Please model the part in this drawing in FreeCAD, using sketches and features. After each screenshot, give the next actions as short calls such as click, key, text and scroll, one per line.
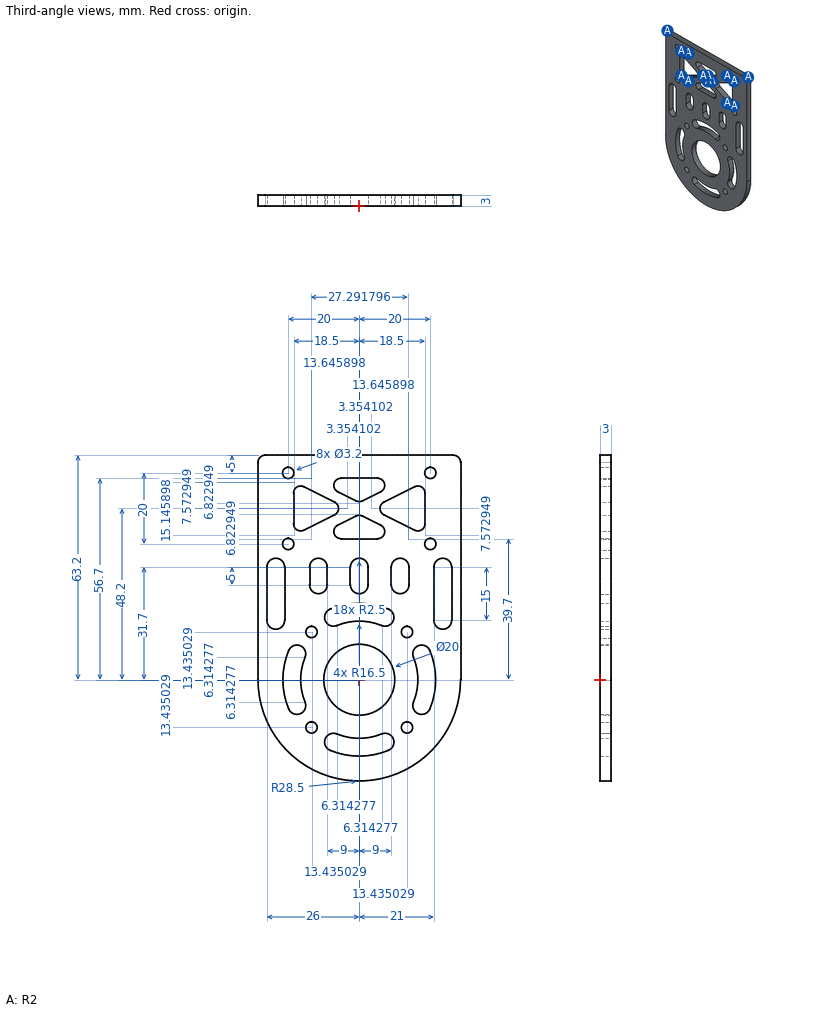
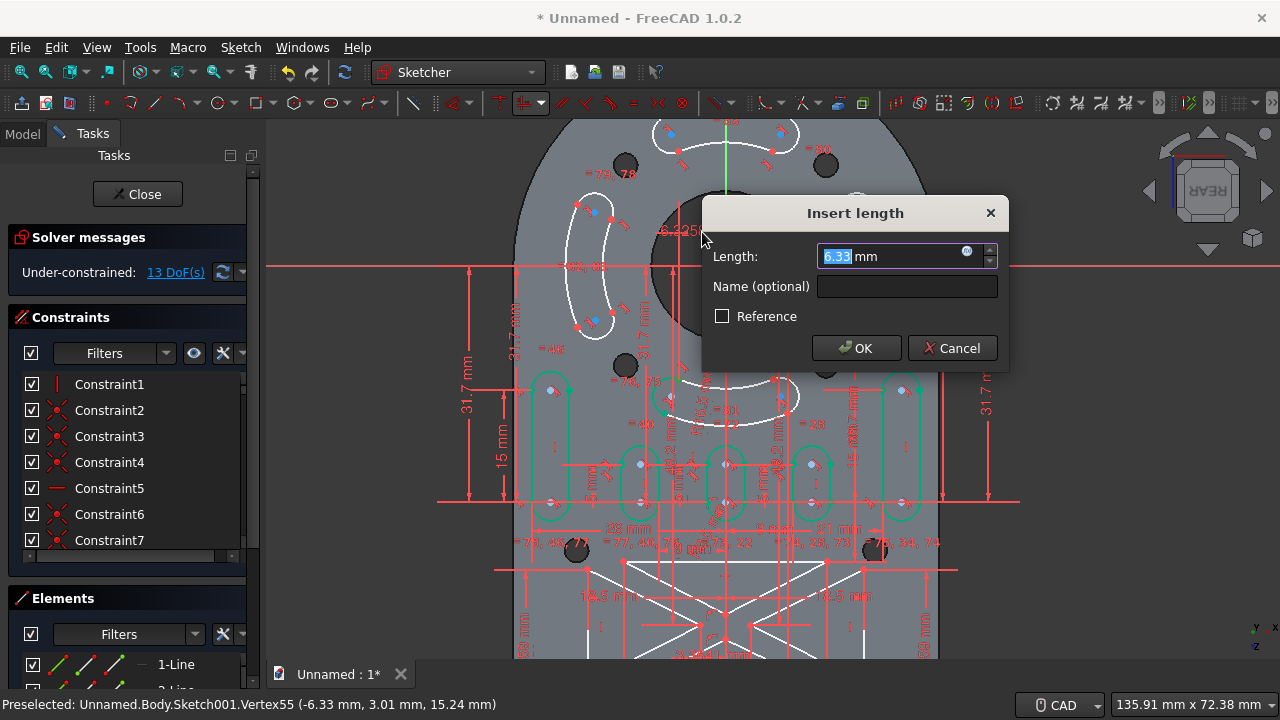
text(6.314277)
key(Return)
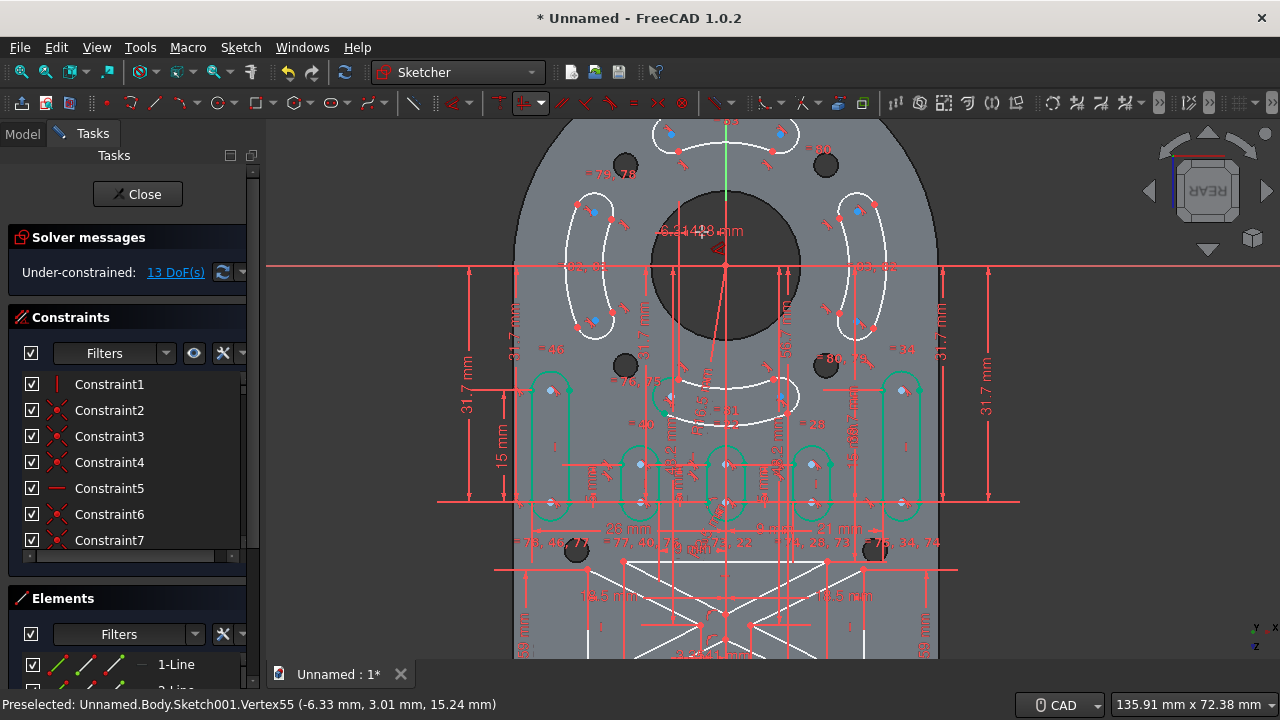
click(773, 379)
click(749, 208)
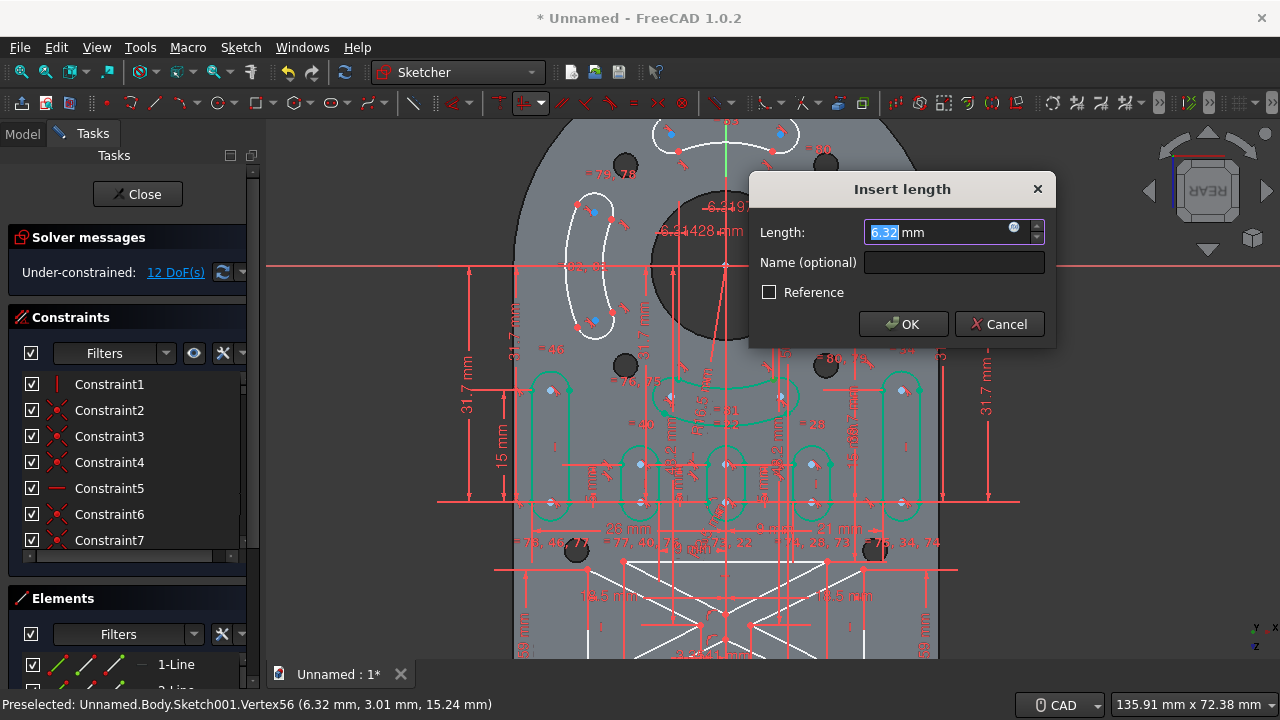
text(6.314277)
key(Return)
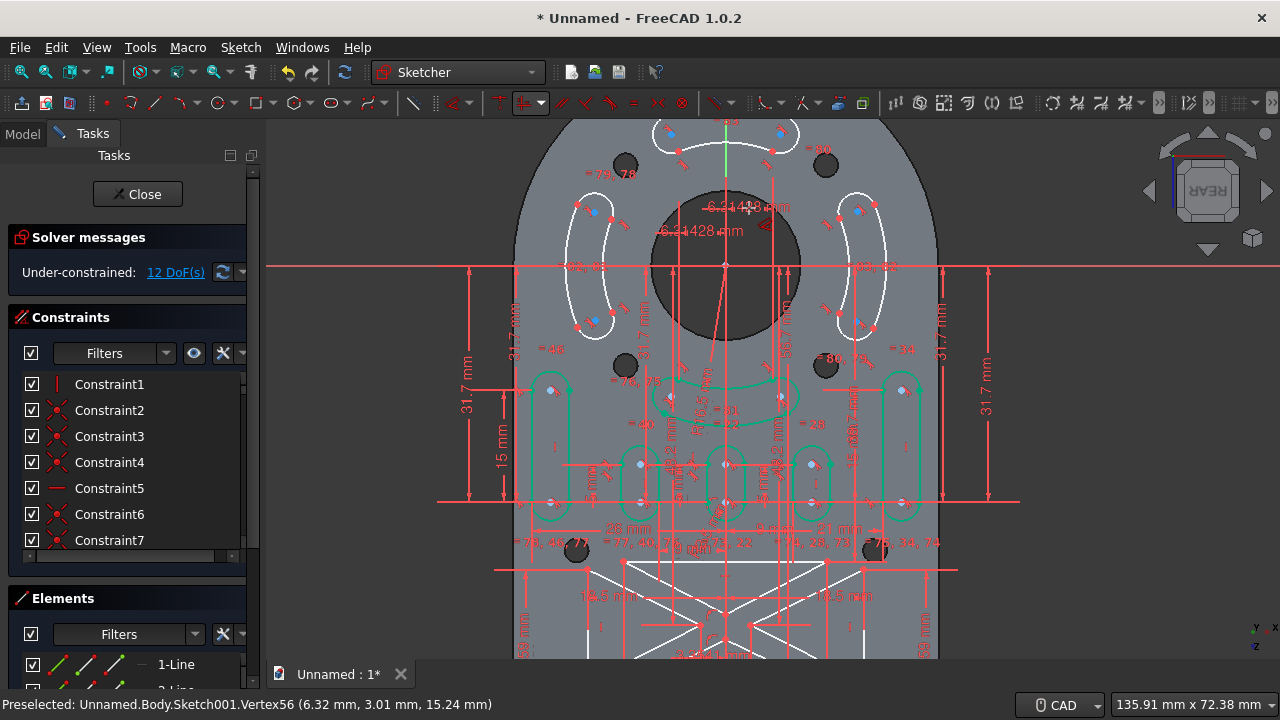
click(612, 219)
click(554, 242)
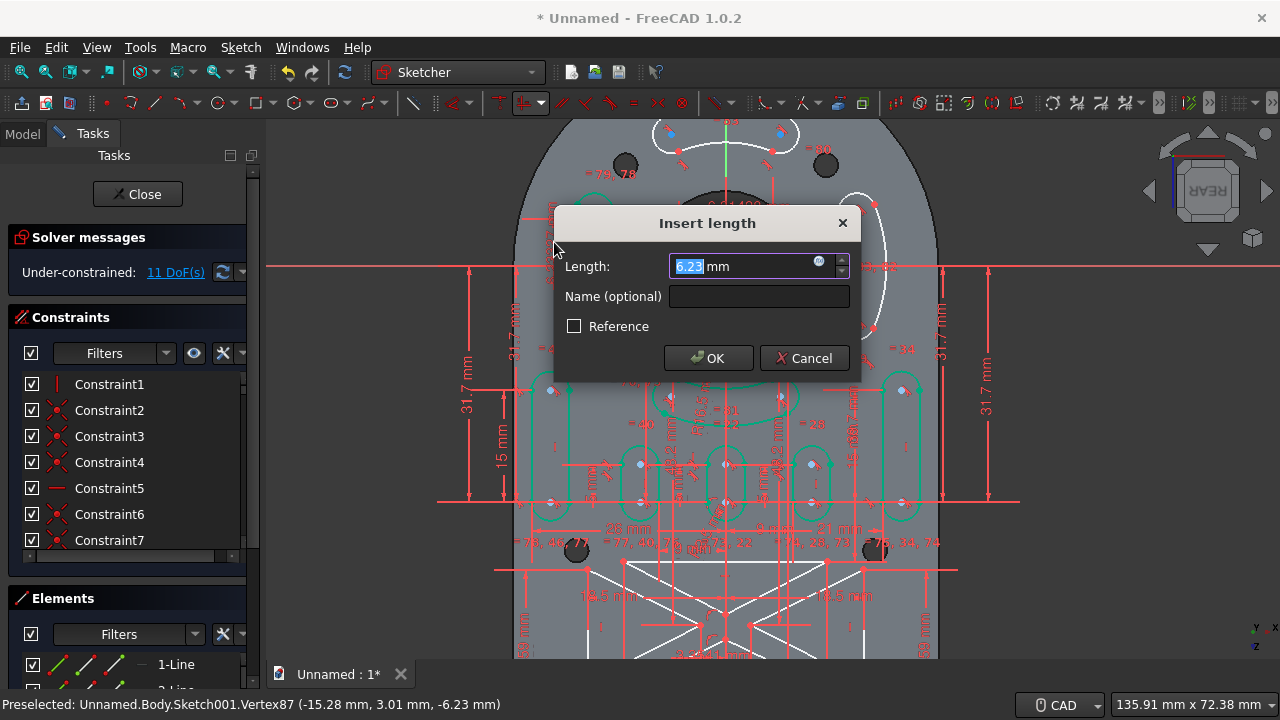
text(6.314277)
key(Return)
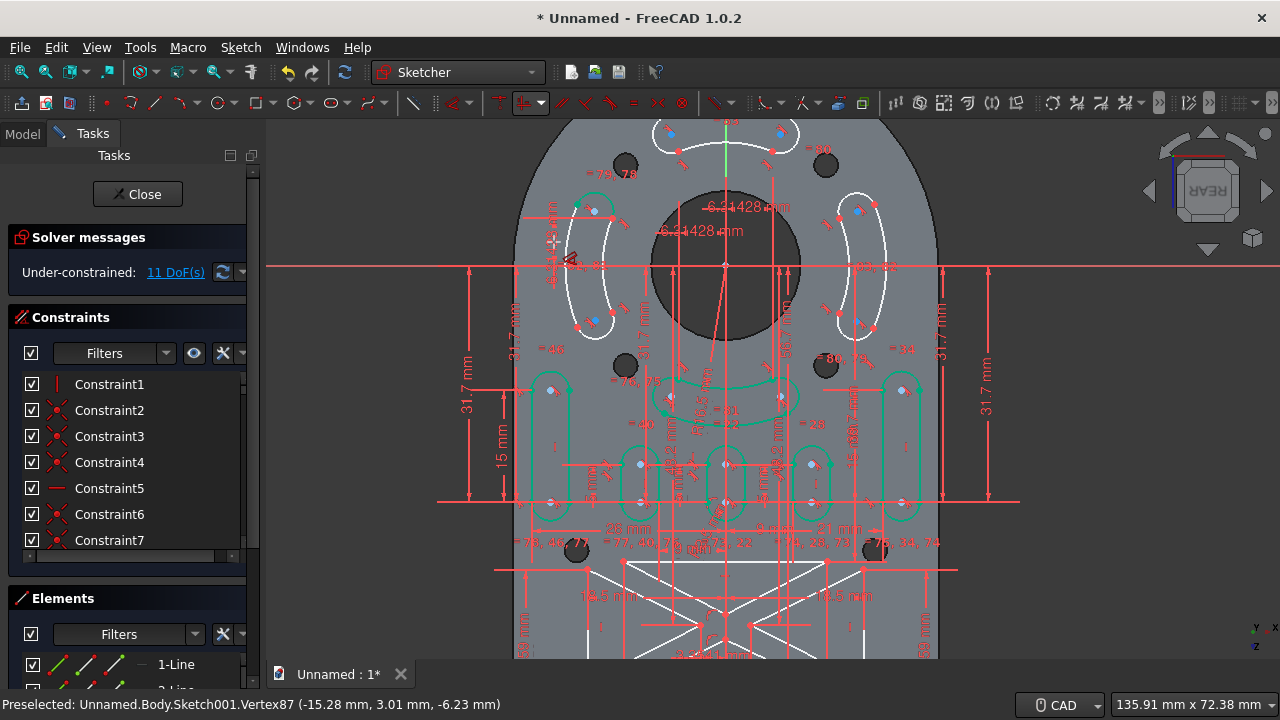
click(612, 313)
click(760, 289)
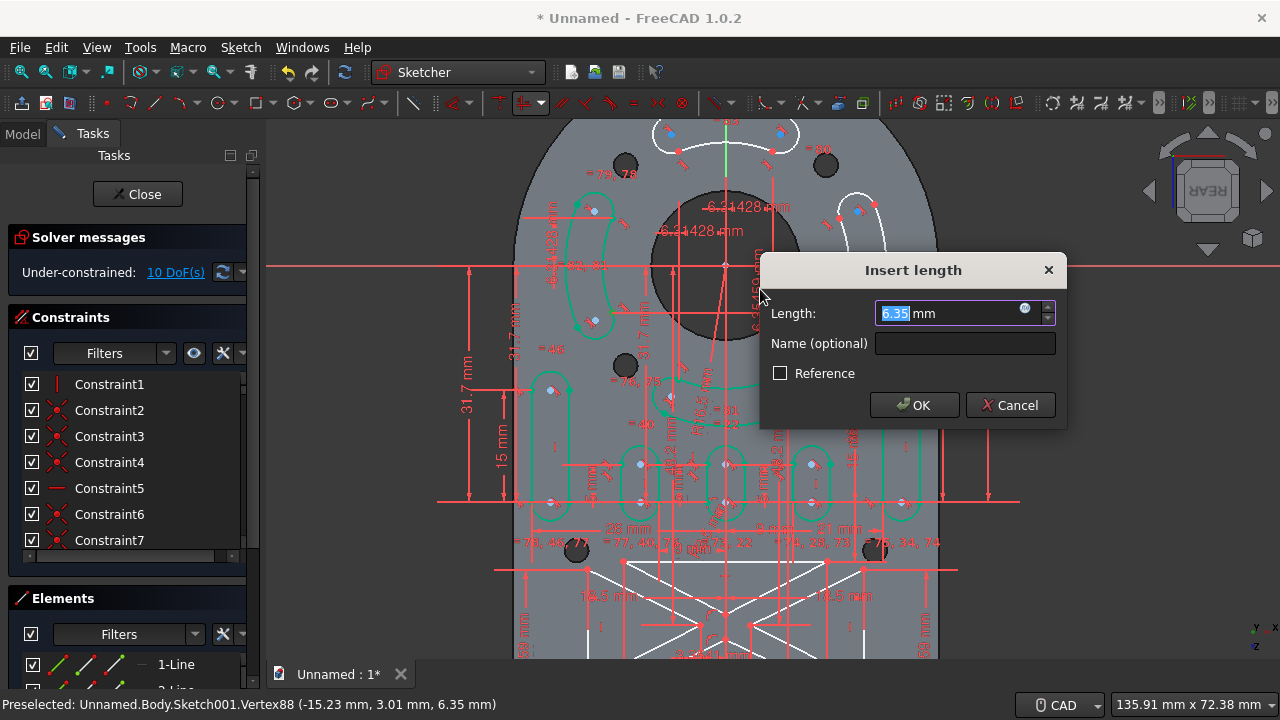
text(6.314277)
key(Return)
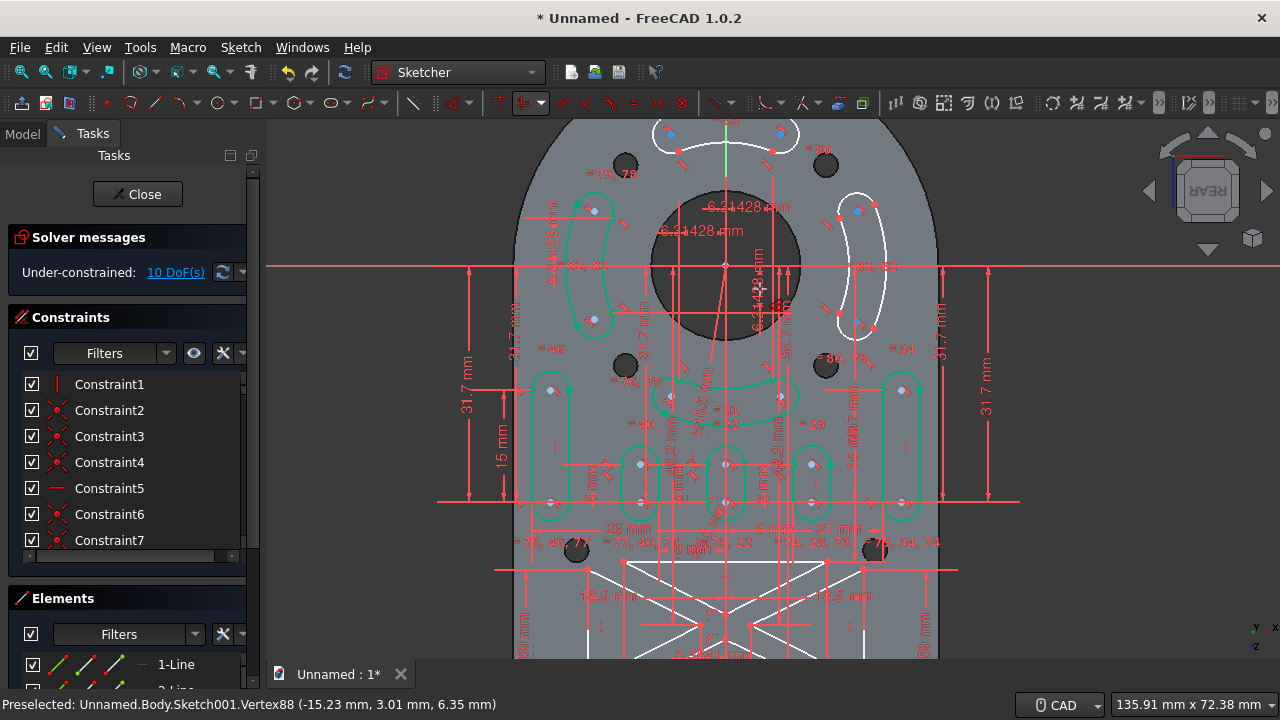
click(839, 314)
click(897, 301)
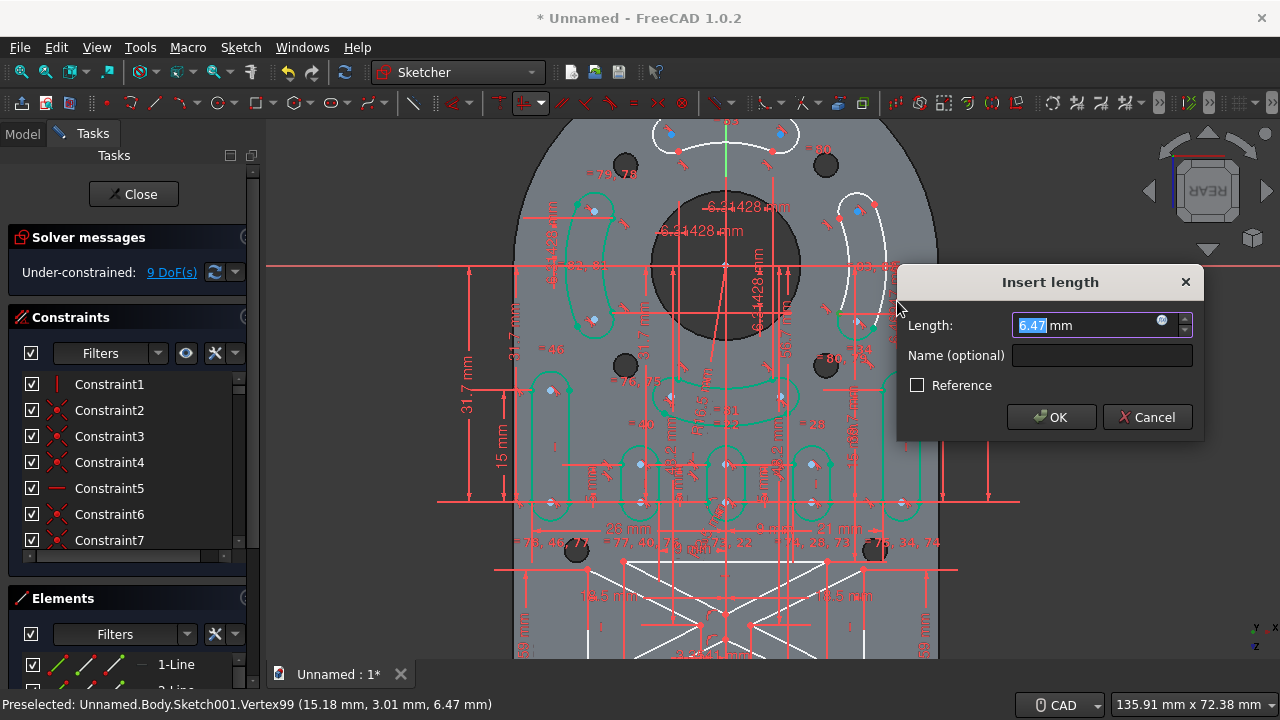
text(6.314277)
key(Return)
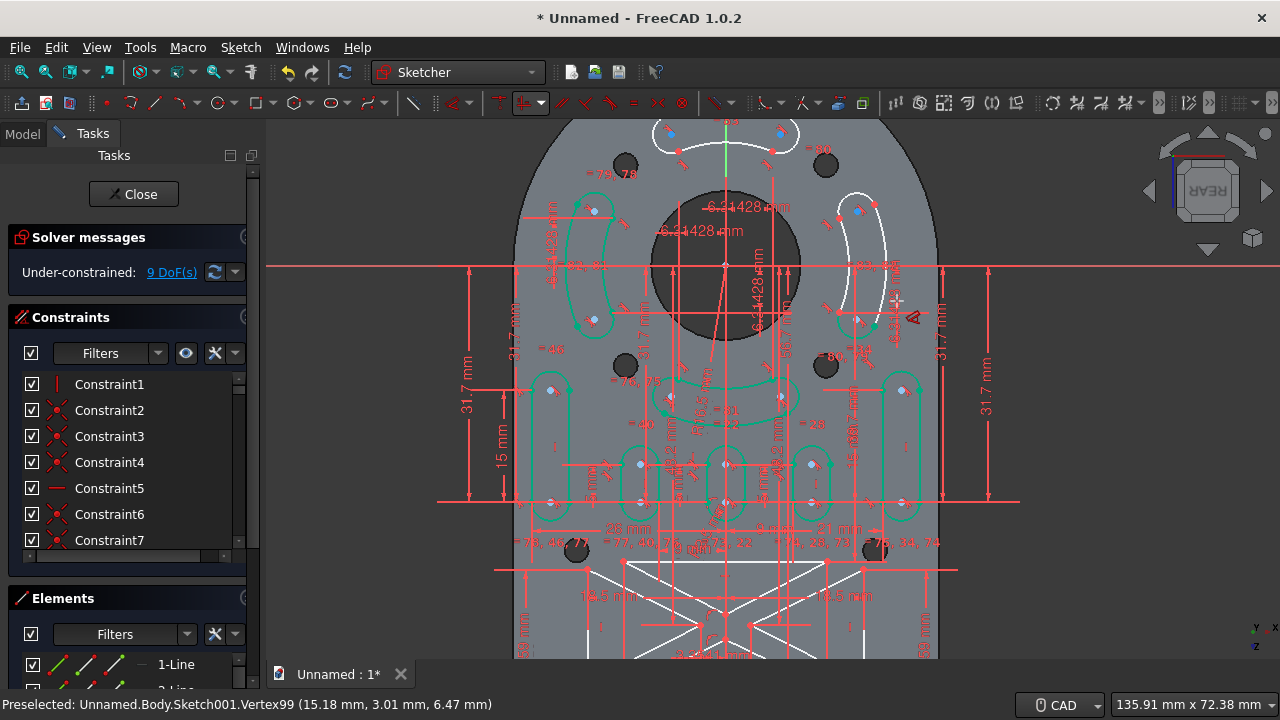
click(840, 219)
click(898, 242)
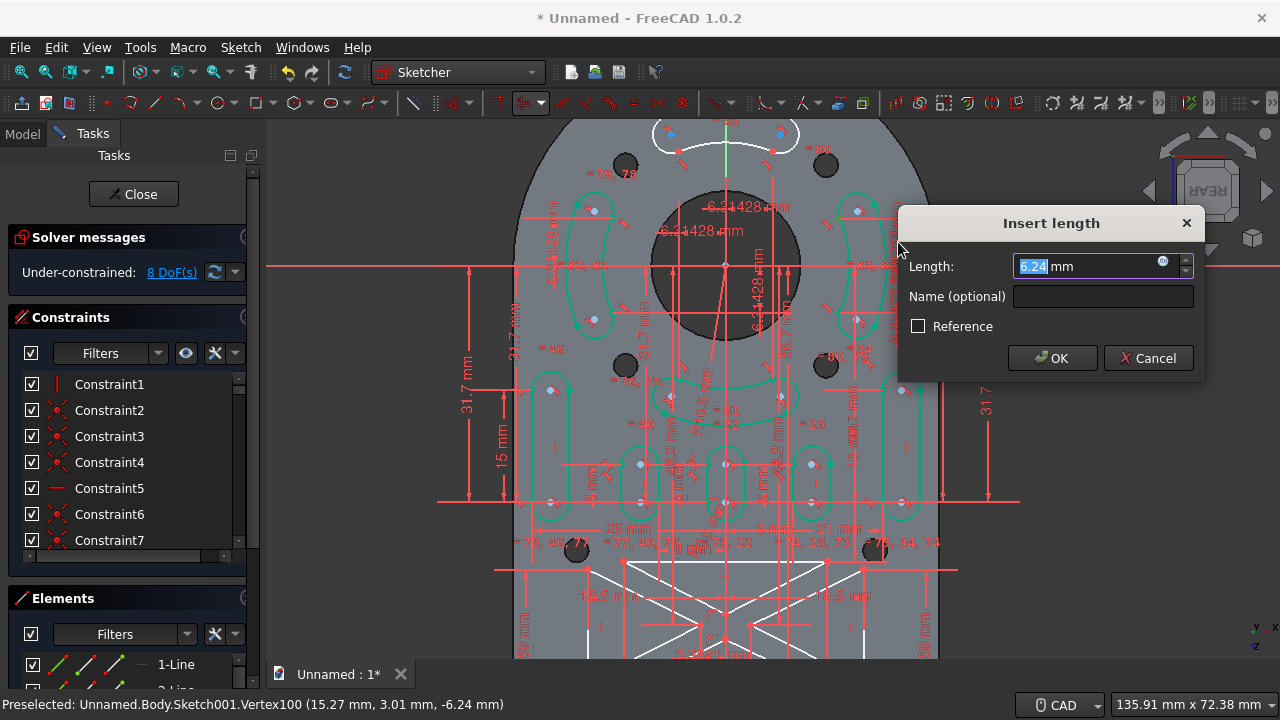
text(6.314277)
key(Return)